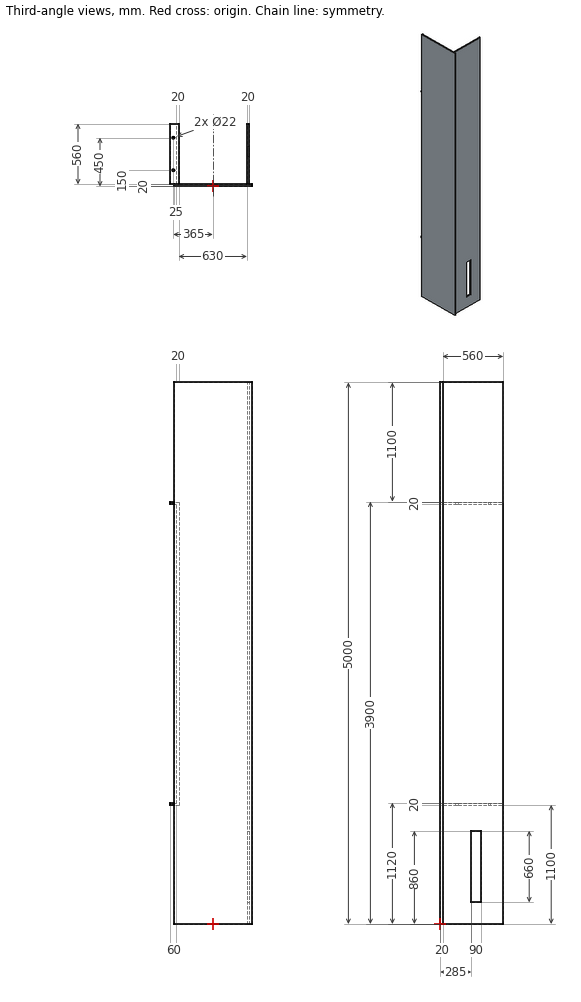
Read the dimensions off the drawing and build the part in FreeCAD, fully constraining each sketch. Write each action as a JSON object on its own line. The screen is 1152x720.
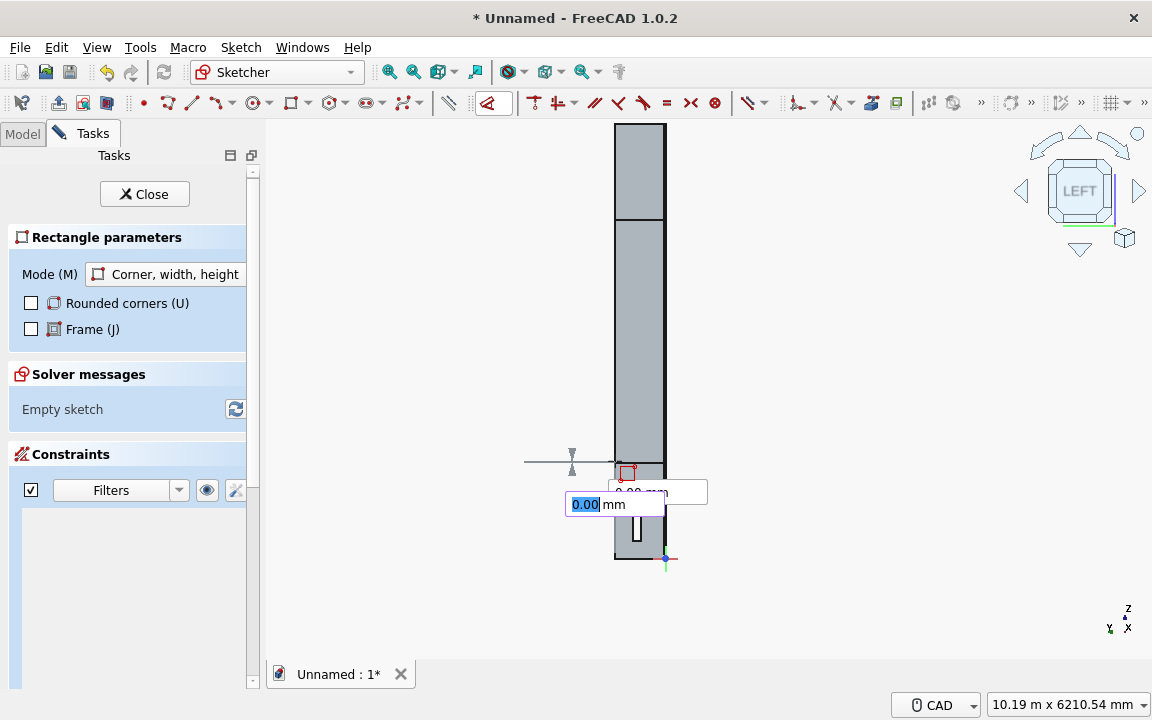
{"action": "scroll", "coordinate": [664, 463], "scroll_direction": "up", "scroll_amount": 12}
{"action": "mouse_move", "coordinate": [659, 459]}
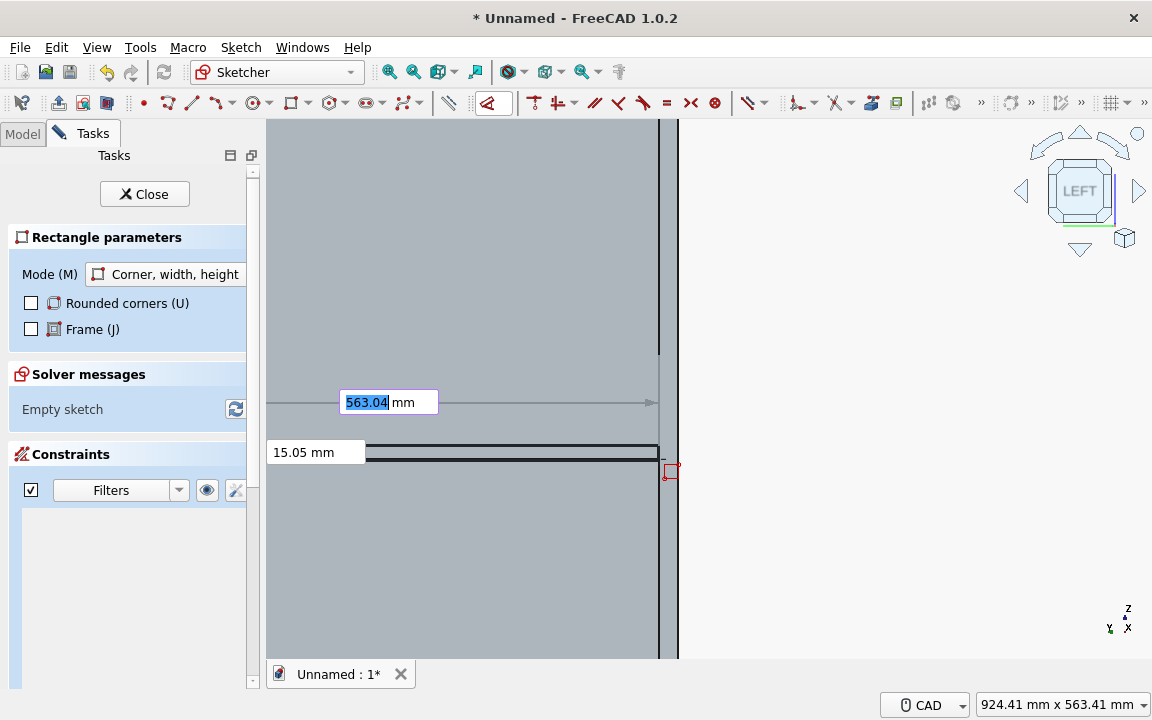
{"action": "type", "text": "560"}
{"action": "key", "text": "Tab"}
{"action": "type", "text": "20"}
{"action": "key", "text": "Return"}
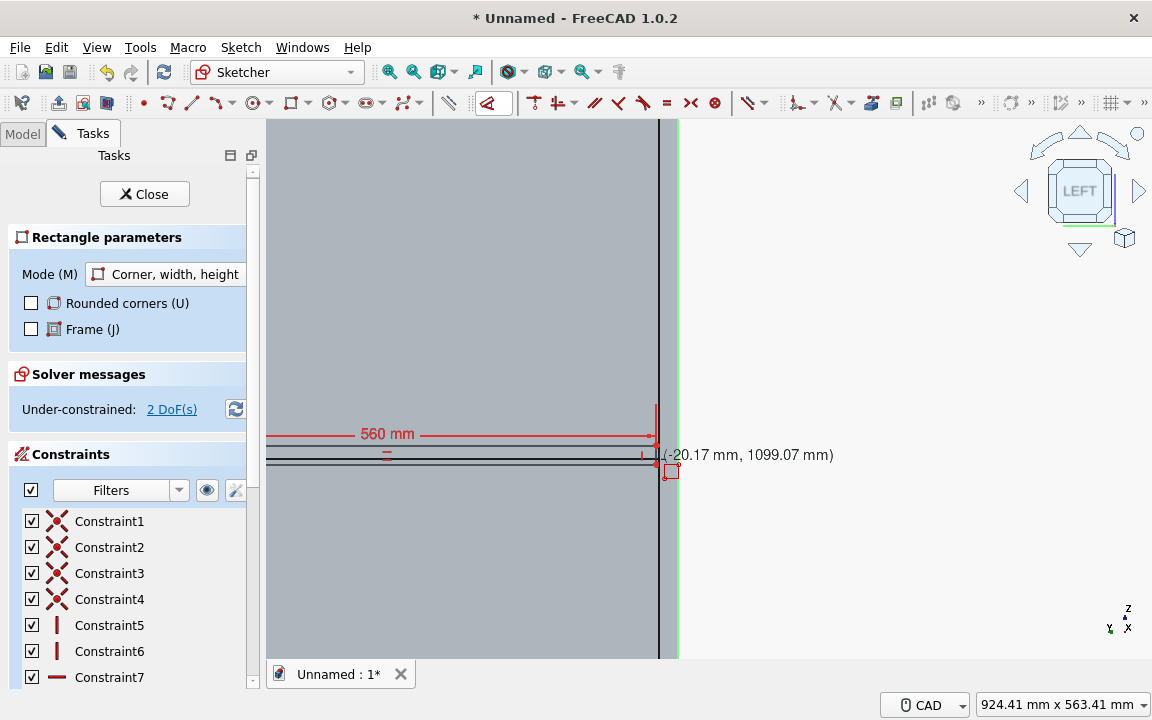
{"action": "scroll", "coordinate": [664, 463], "scroll_direction": "down", "scroll_amount": 12}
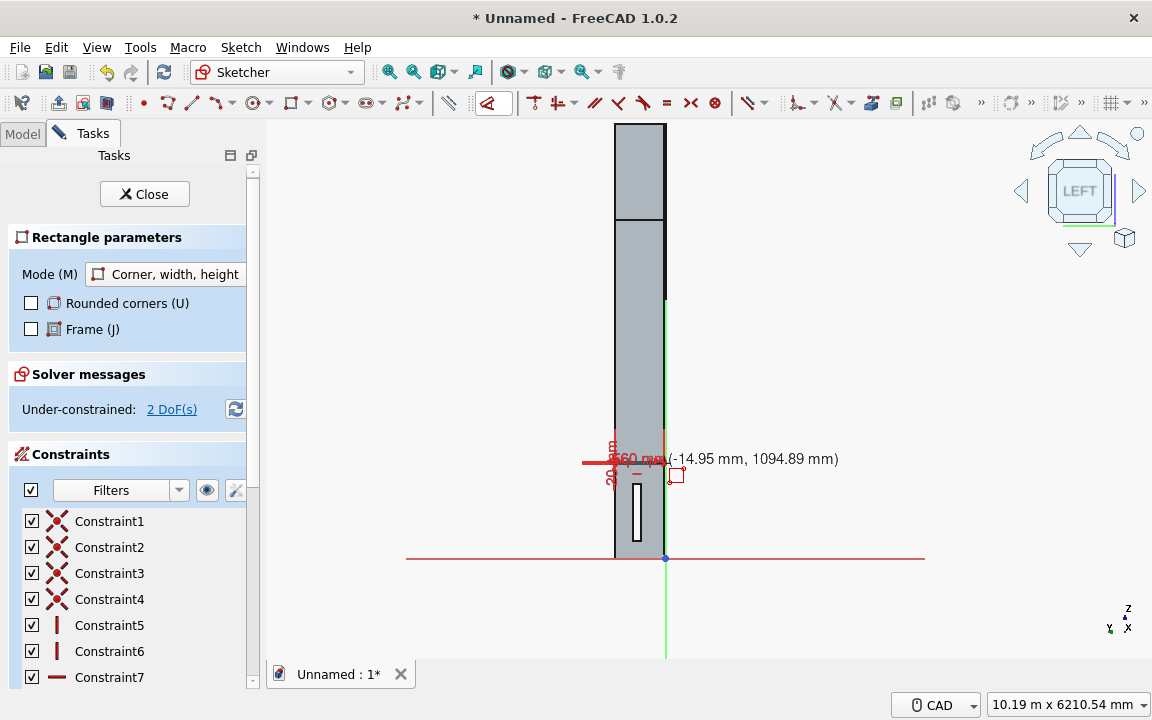
{"action": "scroll", "coordinate": [615, 220], "scroll_direction": "up", "scroll_amount": 12}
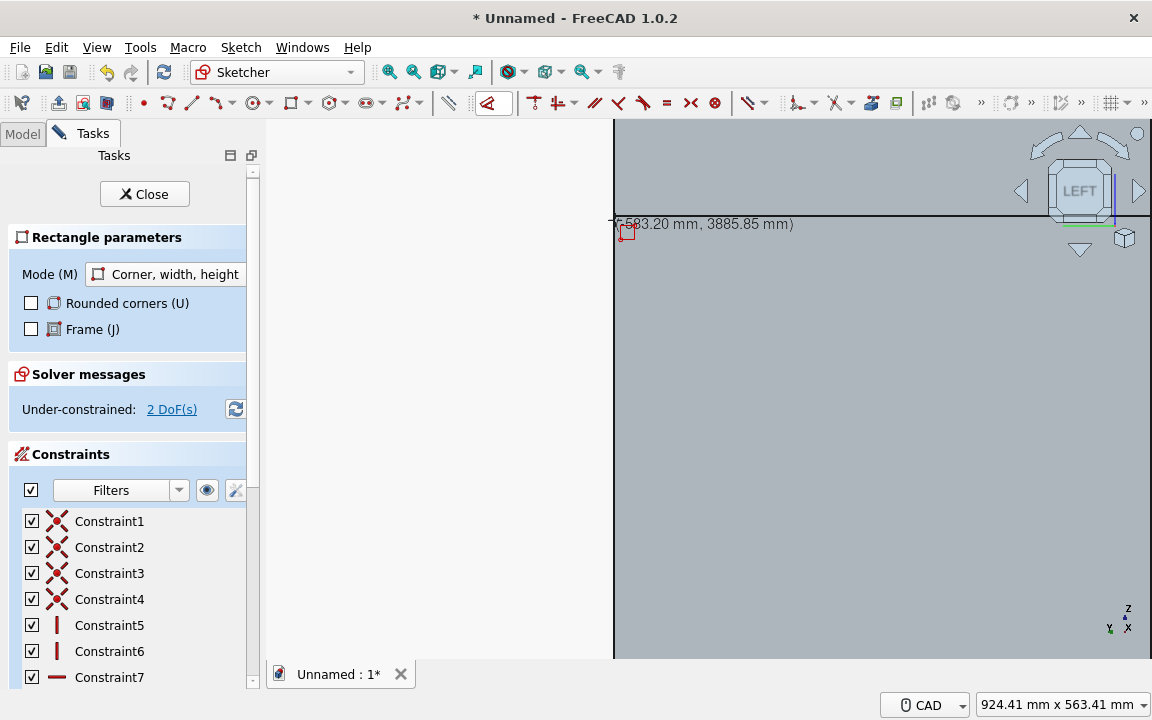
{"action": "scroll", "coordinate": [615, 220], "scroll_direction": "down", "scroll_amount": 12}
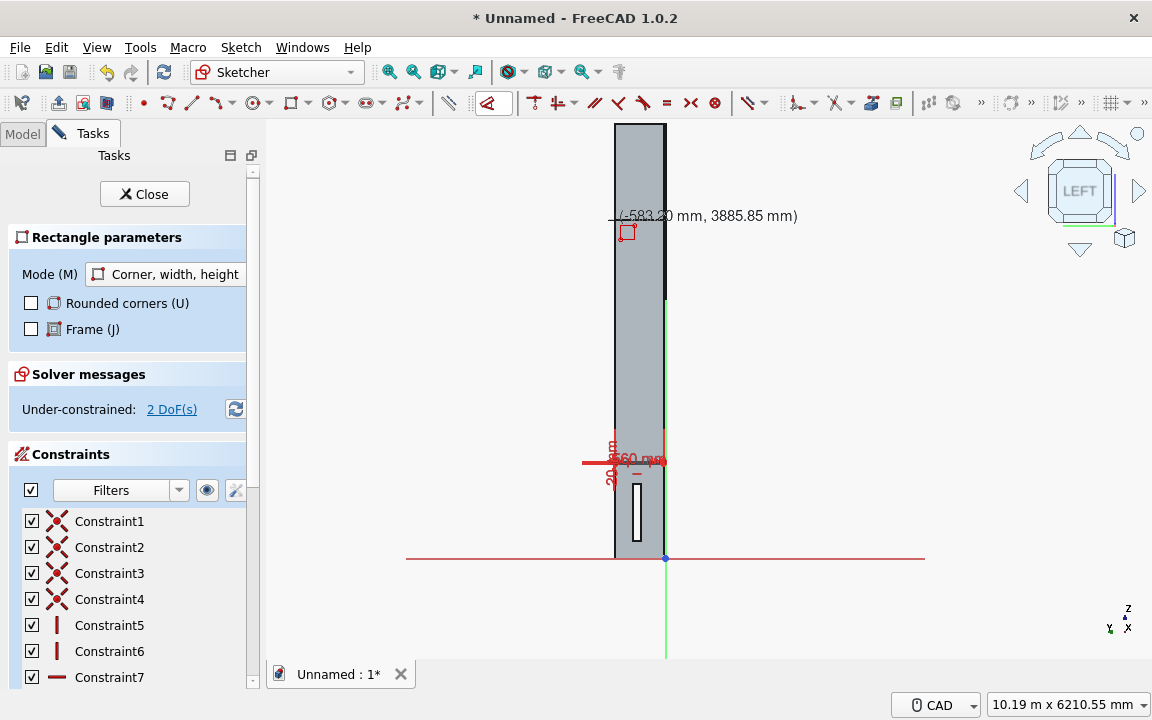
{"action": "left_click", "coordinate": [615, 220]}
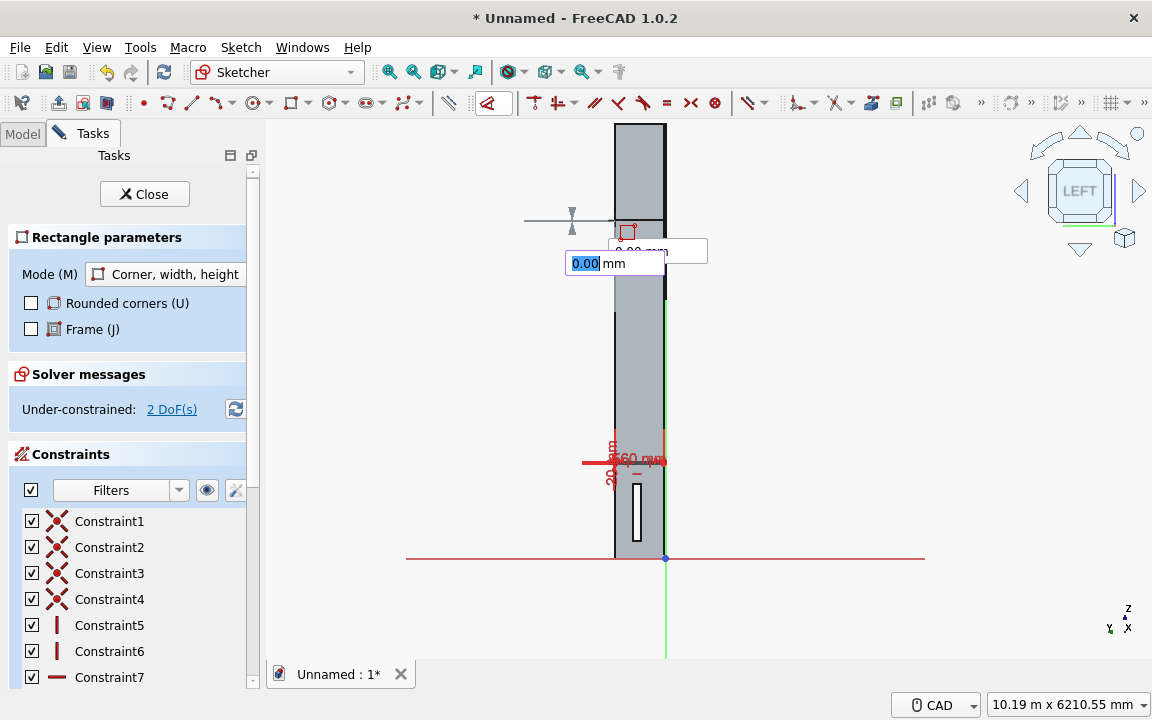
{"action": "scroll", "coordinate": [664, 222], "scroll_direction": "up", "scroll_amount": 12}
{"action": "mouse_move", "coordinate": [659, 215]}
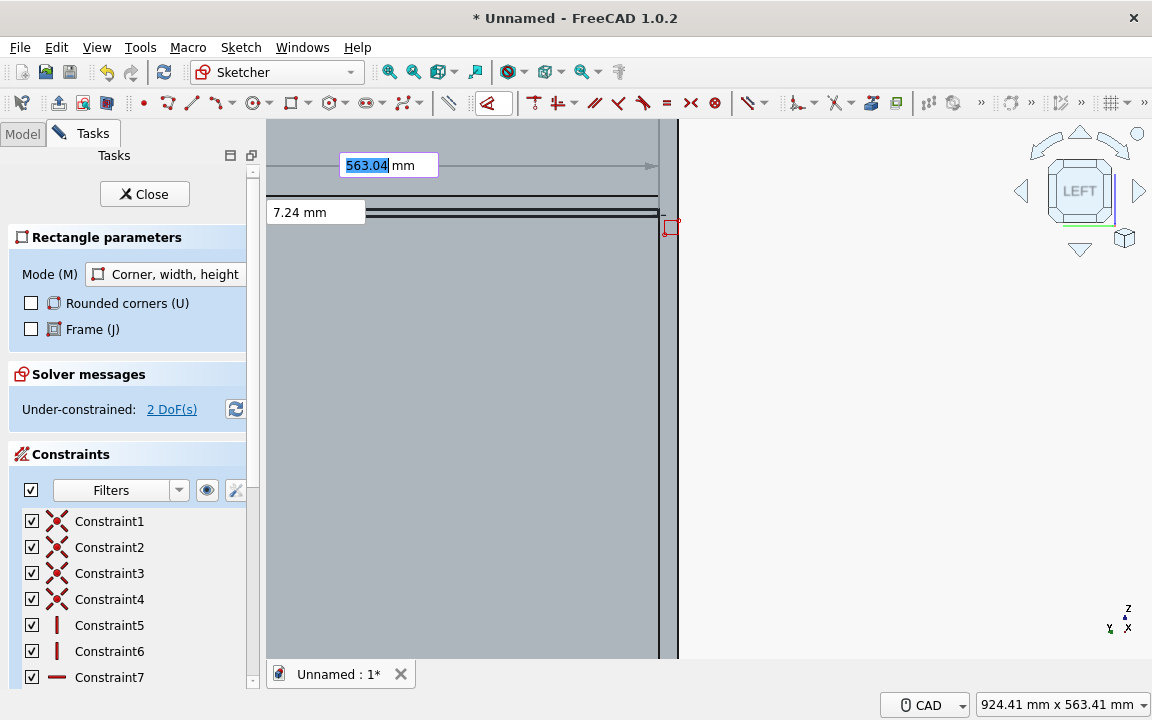
{"action": "type", "text": "560"}
{"action": "key", "text": "Tab"}
{"action": "type", "text": "20"}
{"action": "key", "text": "Return"}
{"action": "key", "text": "Escape"}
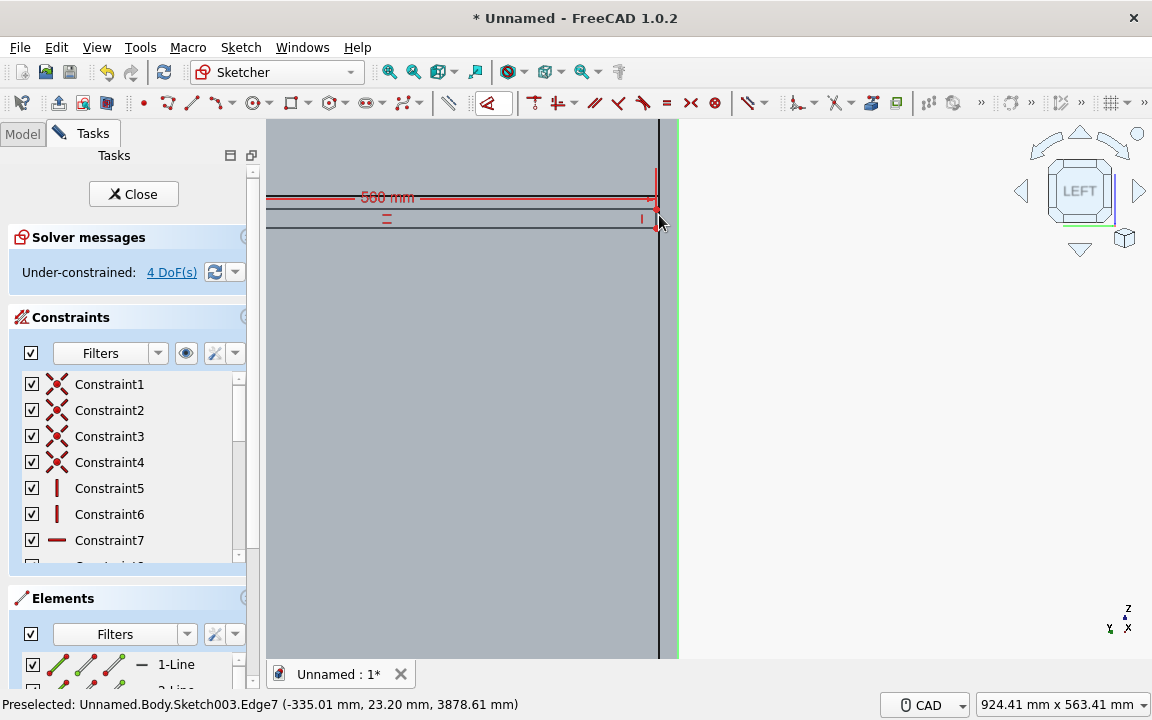
{"action": "scroll", "coordinate": [664, 222], "scroll_direction": "down", "scroll_amount": 12}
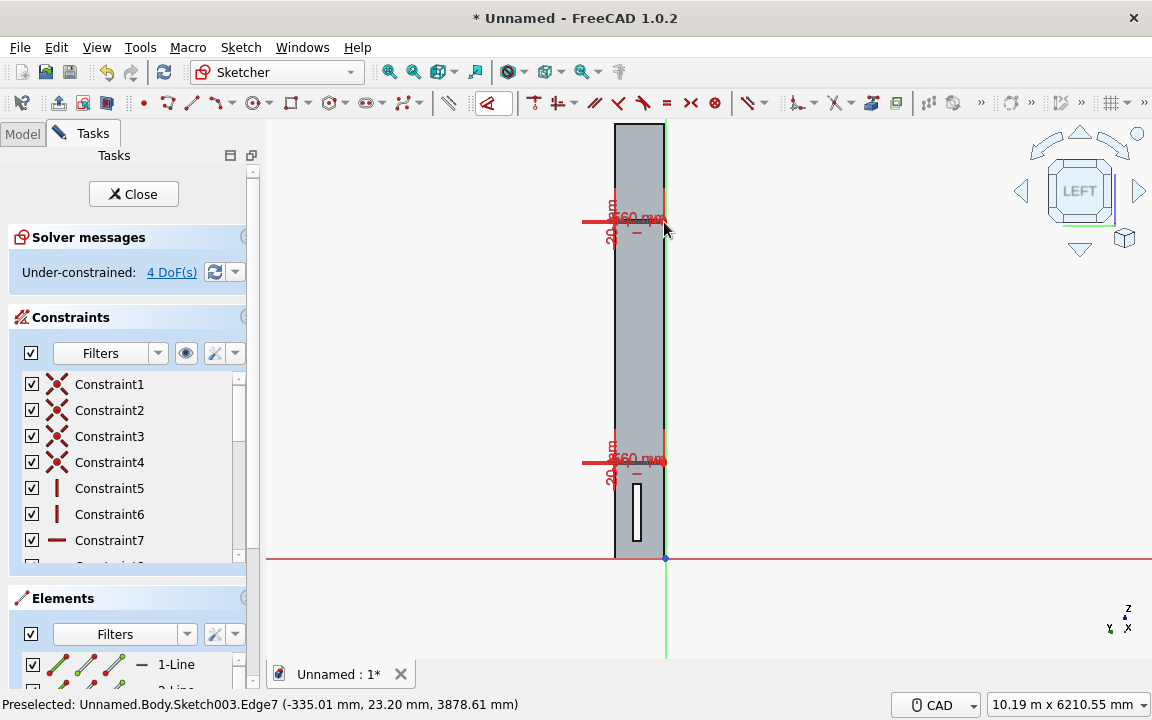
{"action": "scroll", "coordinate": [664, 464], "scroll_direction": "up", "scroll_amount": 16}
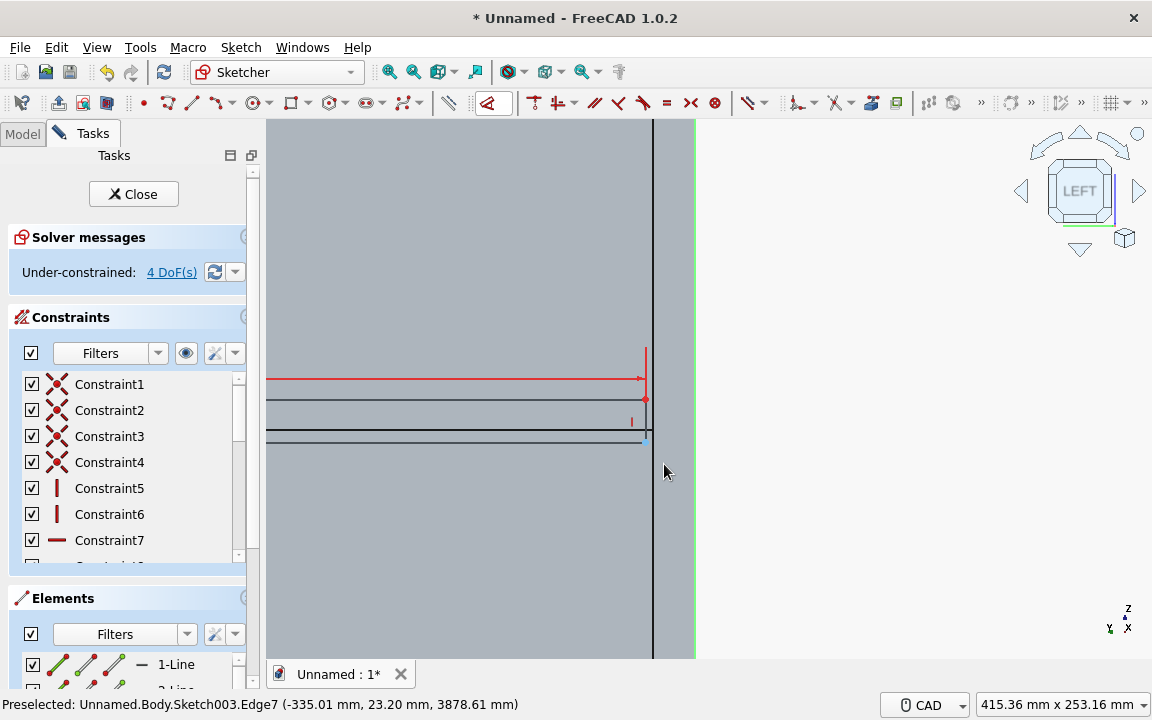
{"action": "left_click", "coordinate": [646, 443]}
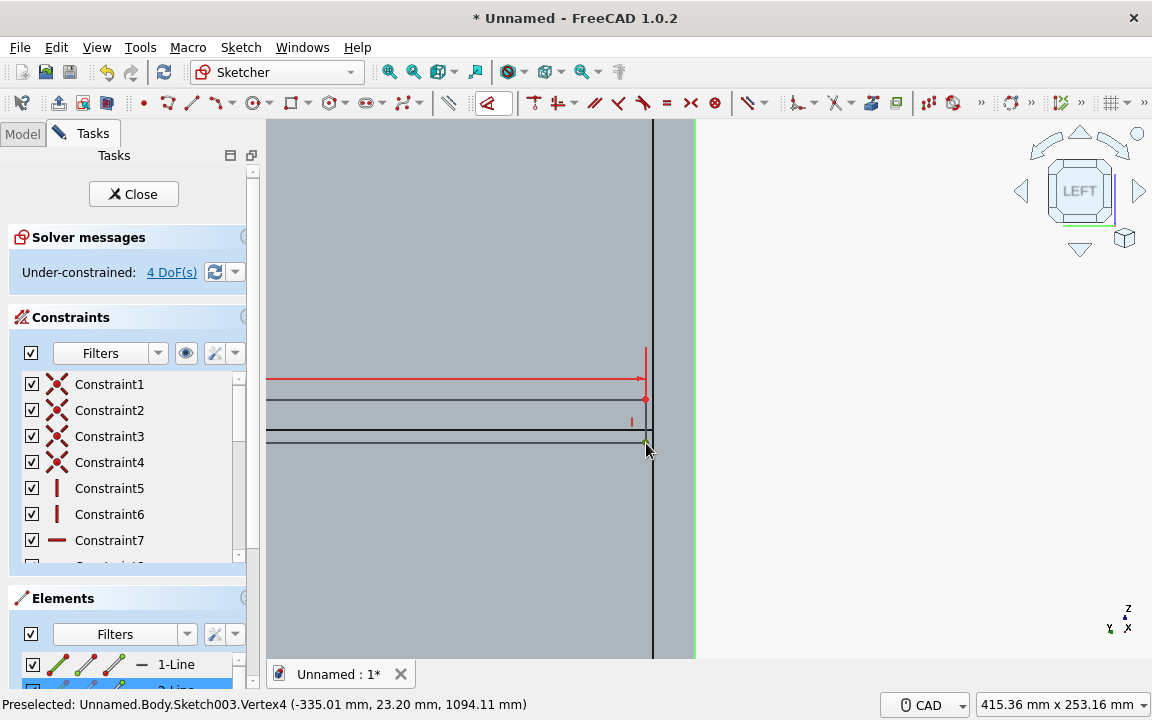
{"action": "left_click", "coordinate": [506, 104]}